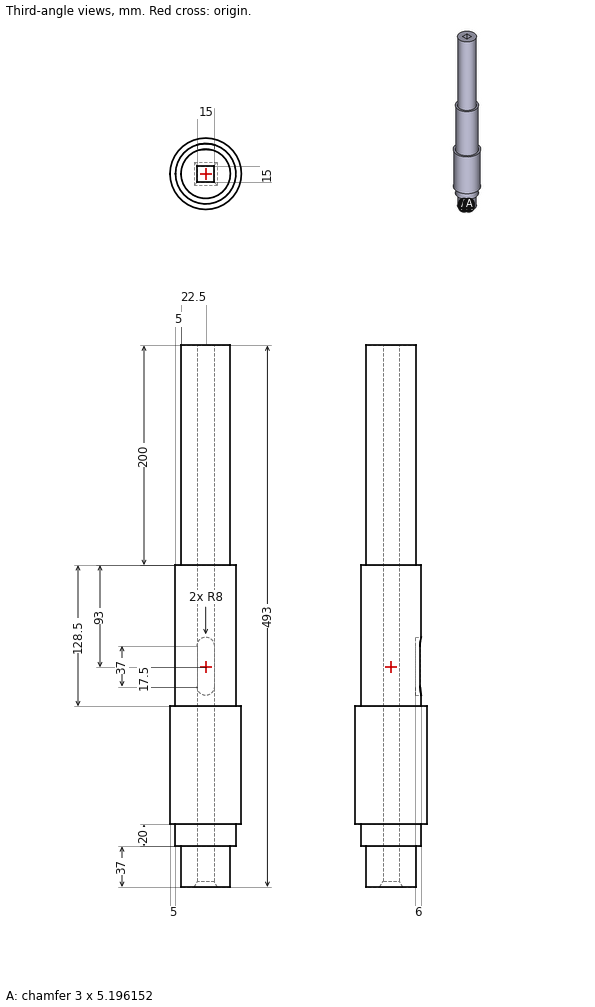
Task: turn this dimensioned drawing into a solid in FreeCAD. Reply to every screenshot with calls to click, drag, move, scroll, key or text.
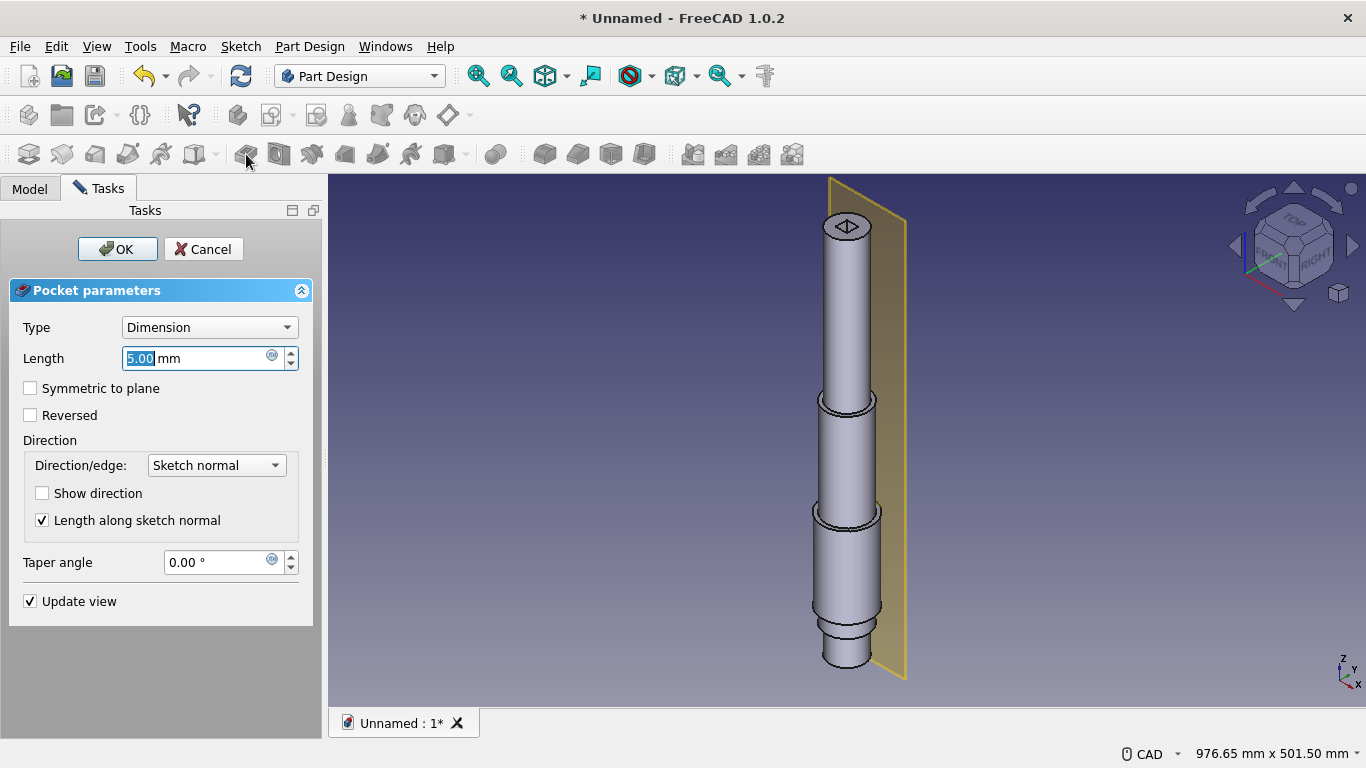
text(6)
key(Tab)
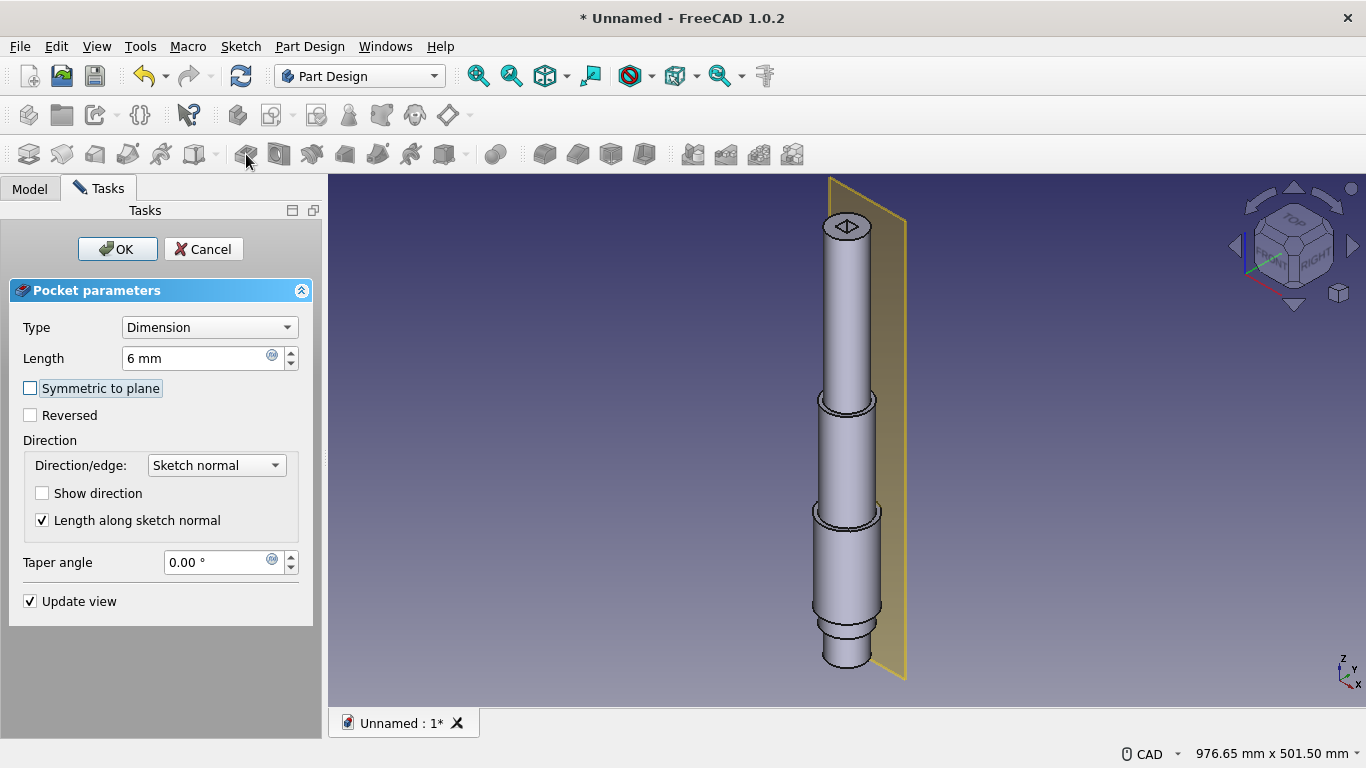
click(31, 415)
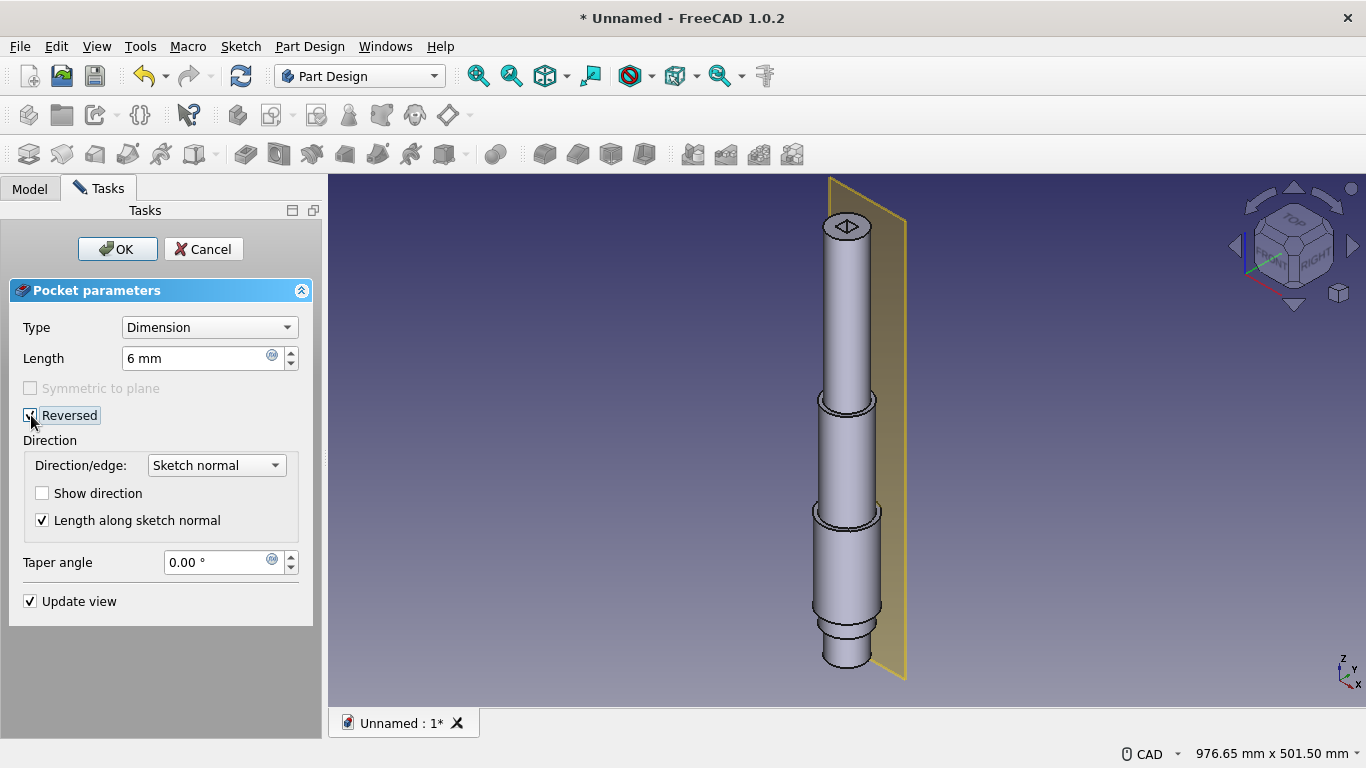
click(118, 249)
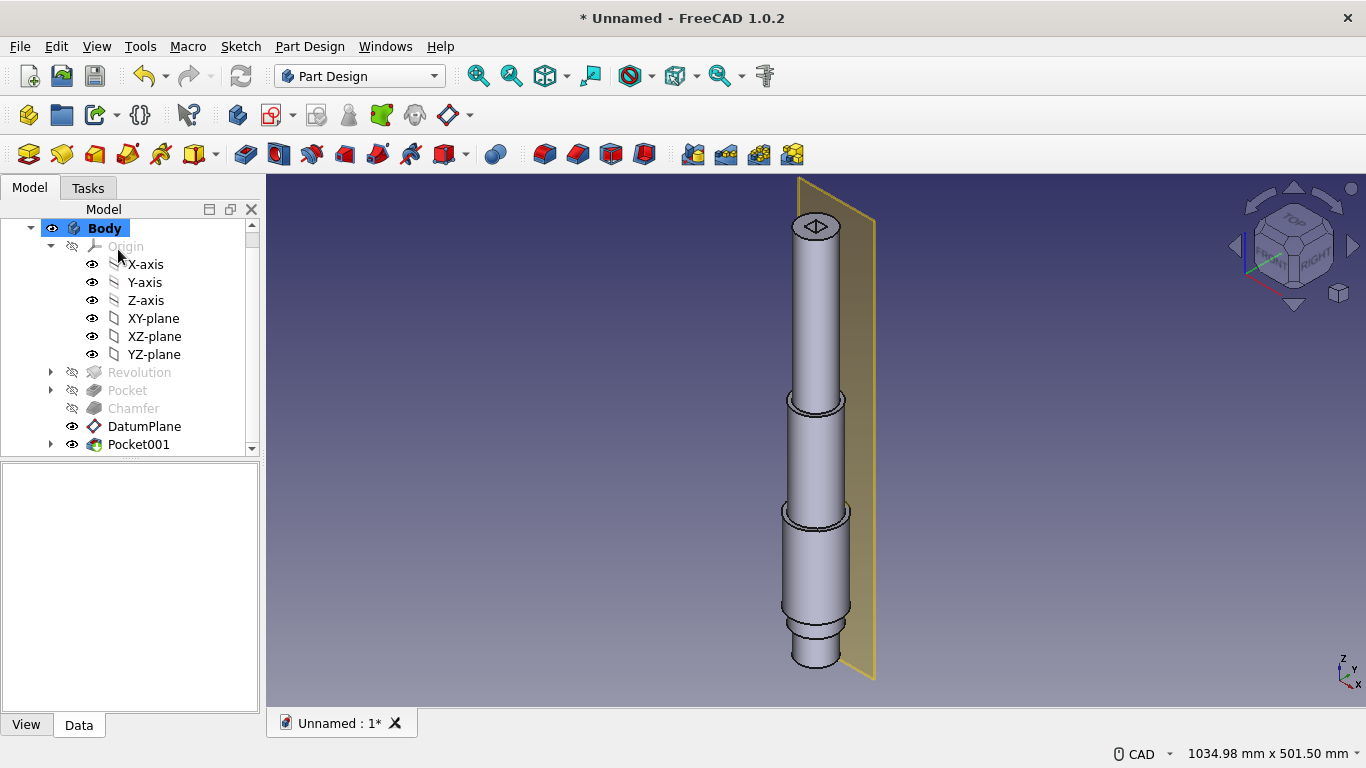
click(117, 426)
key(space)